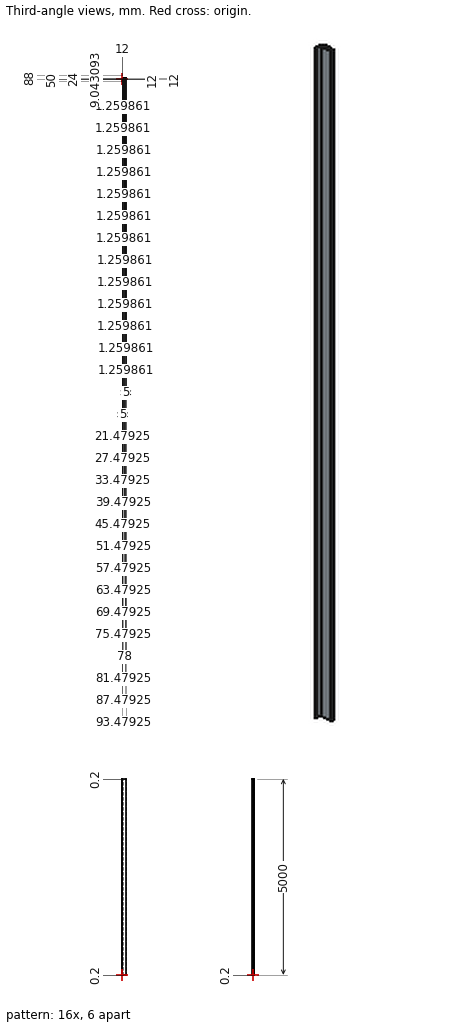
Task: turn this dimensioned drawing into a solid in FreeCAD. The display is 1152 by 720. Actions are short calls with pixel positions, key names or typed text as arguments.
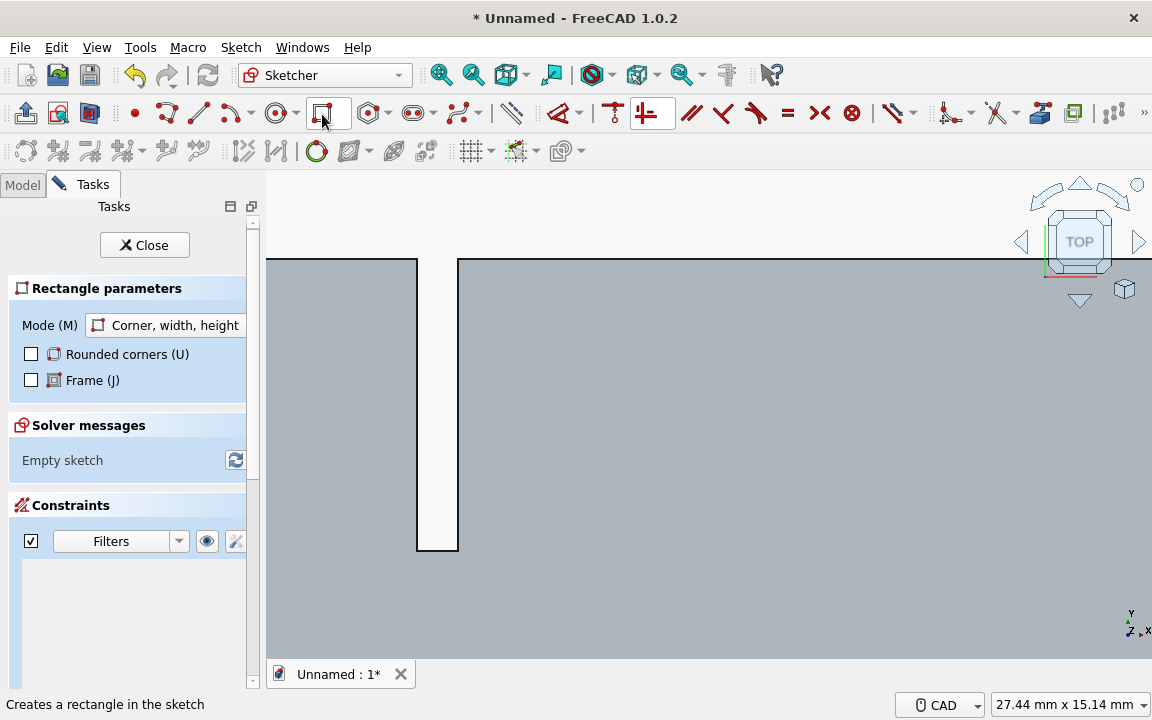
click(611, 259)
click(652, 551)
key(Escape)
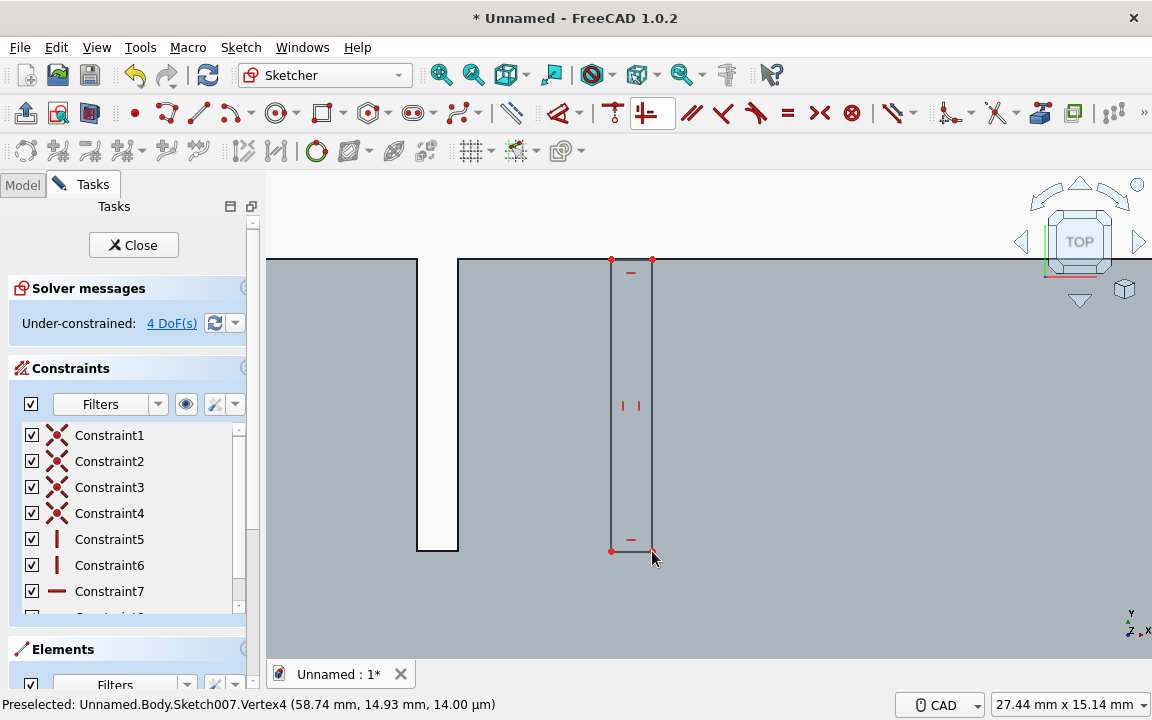
click(558, 114)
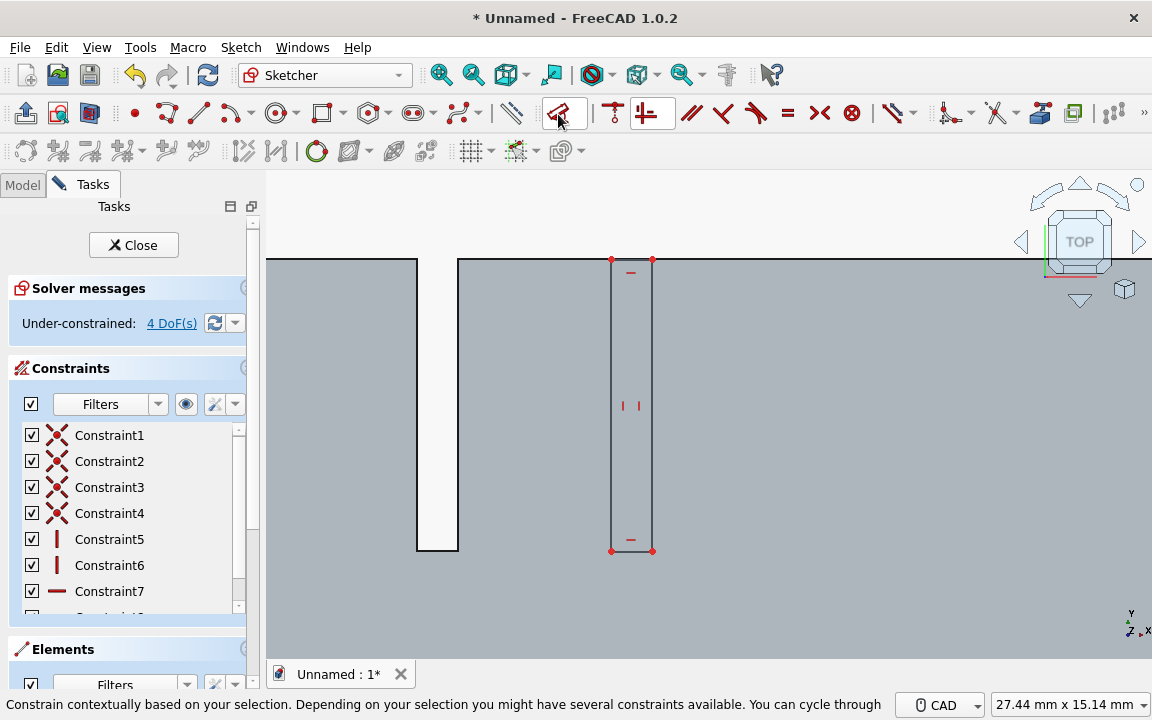
click(611, 260)
click(645, 575)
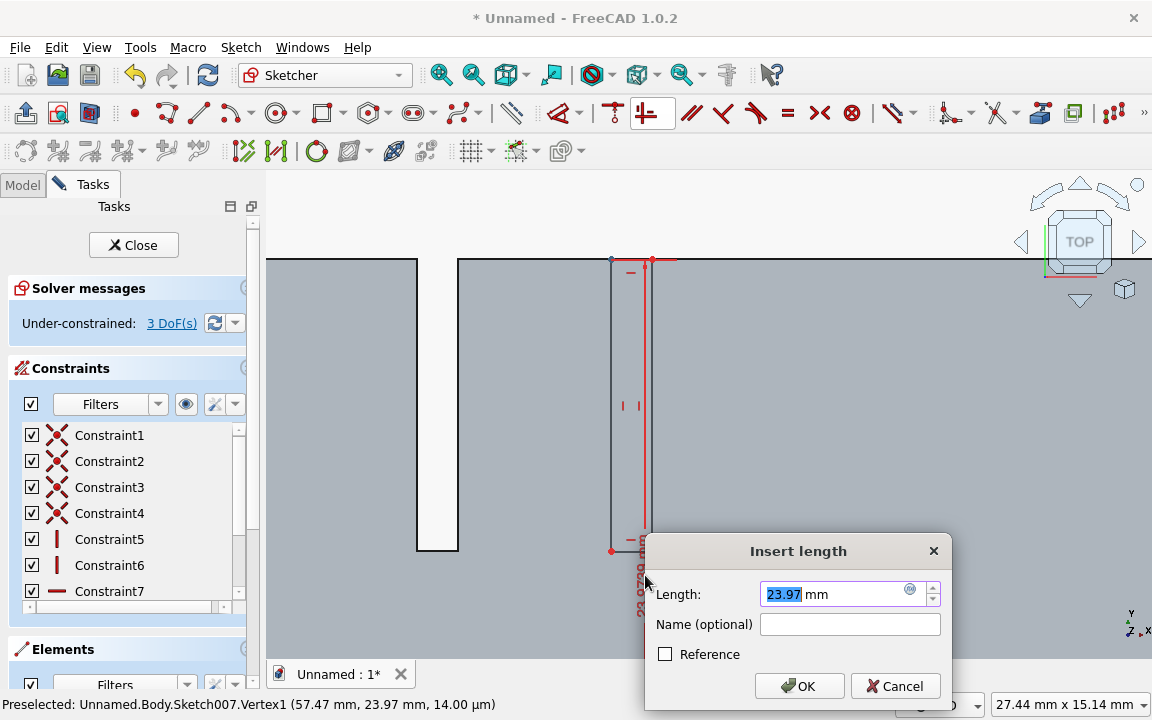
text(24)
key(Return)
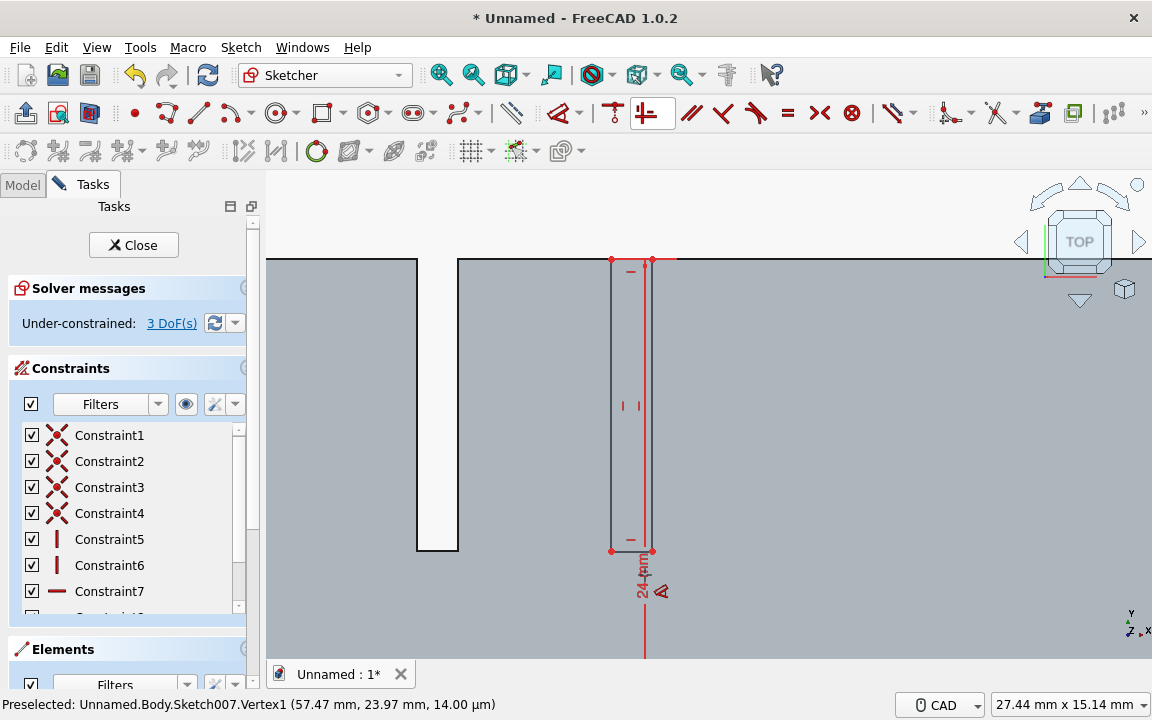
click(611, 347)
click(577, 406)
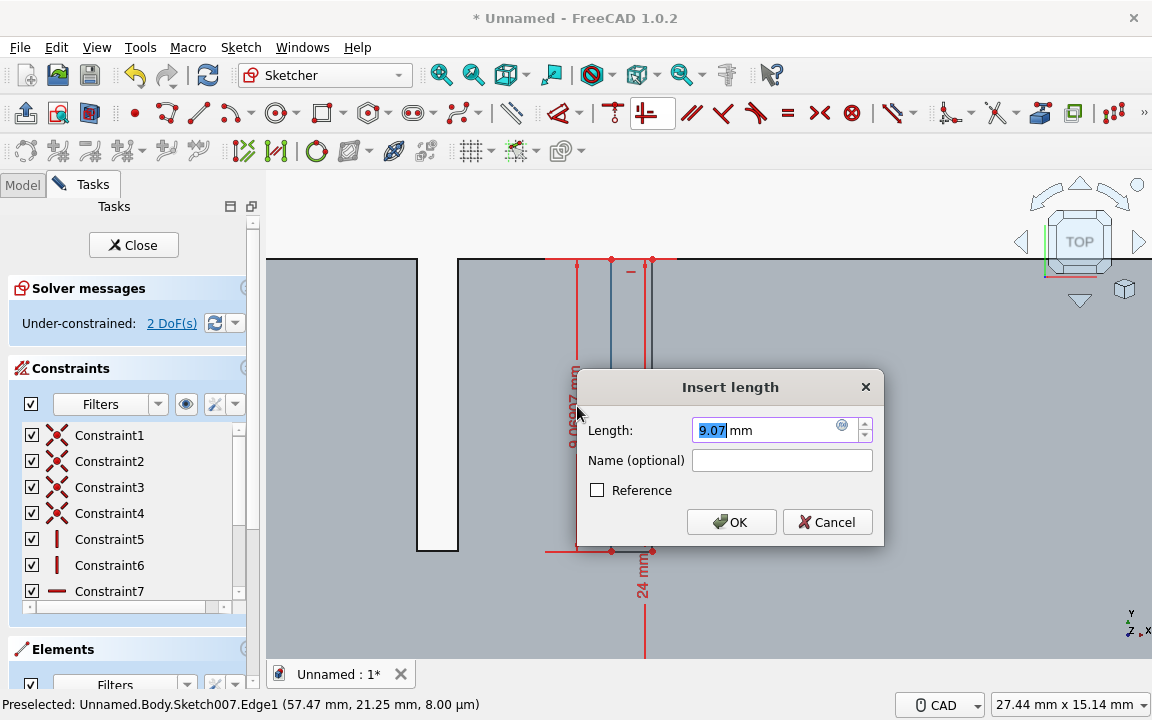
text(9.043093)
key(Return)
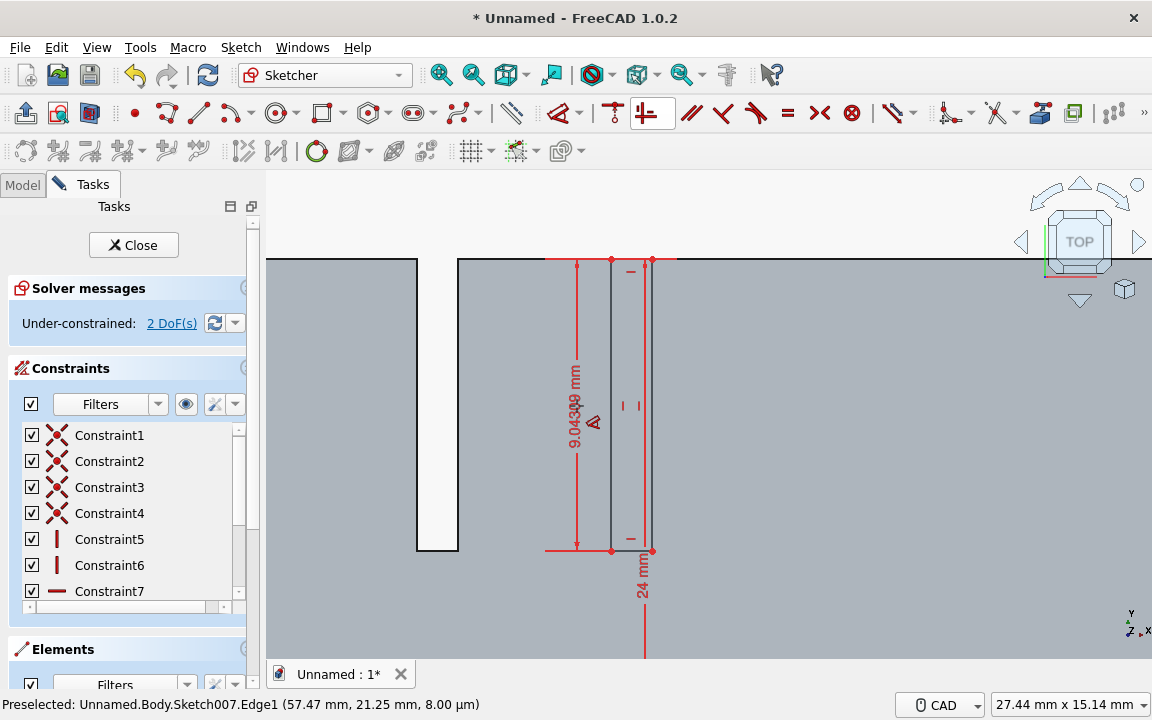
click(623, 551)
click(631, 517)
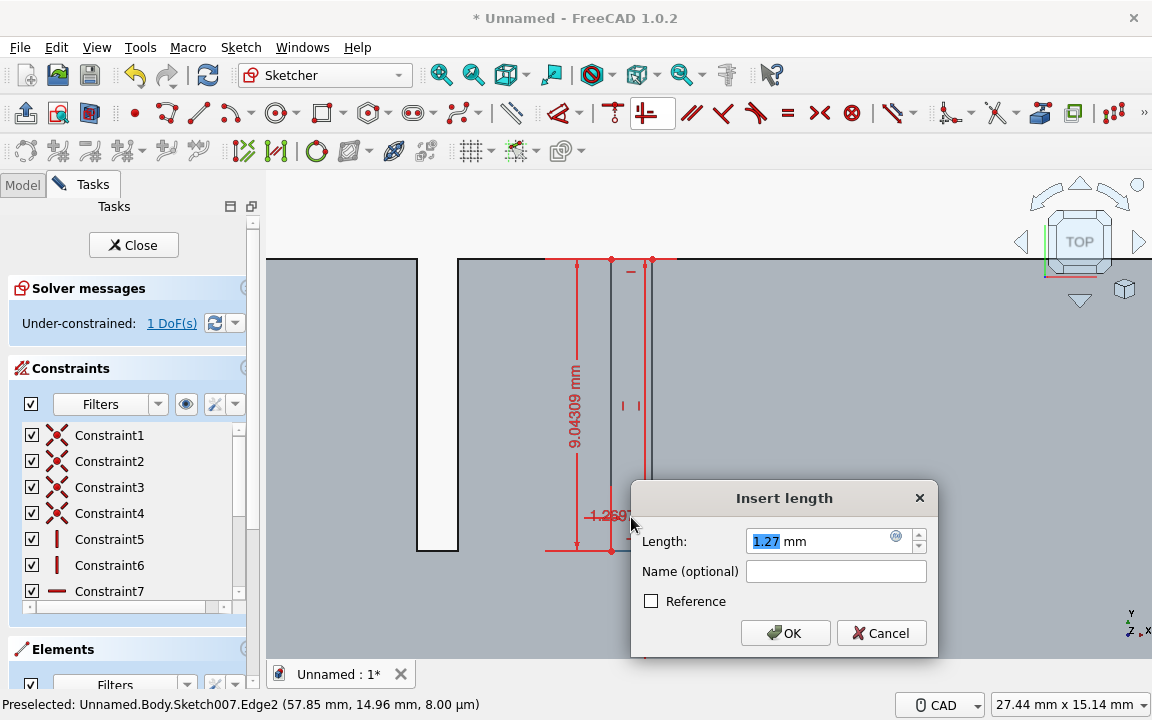
text(1.259861)
key(Return)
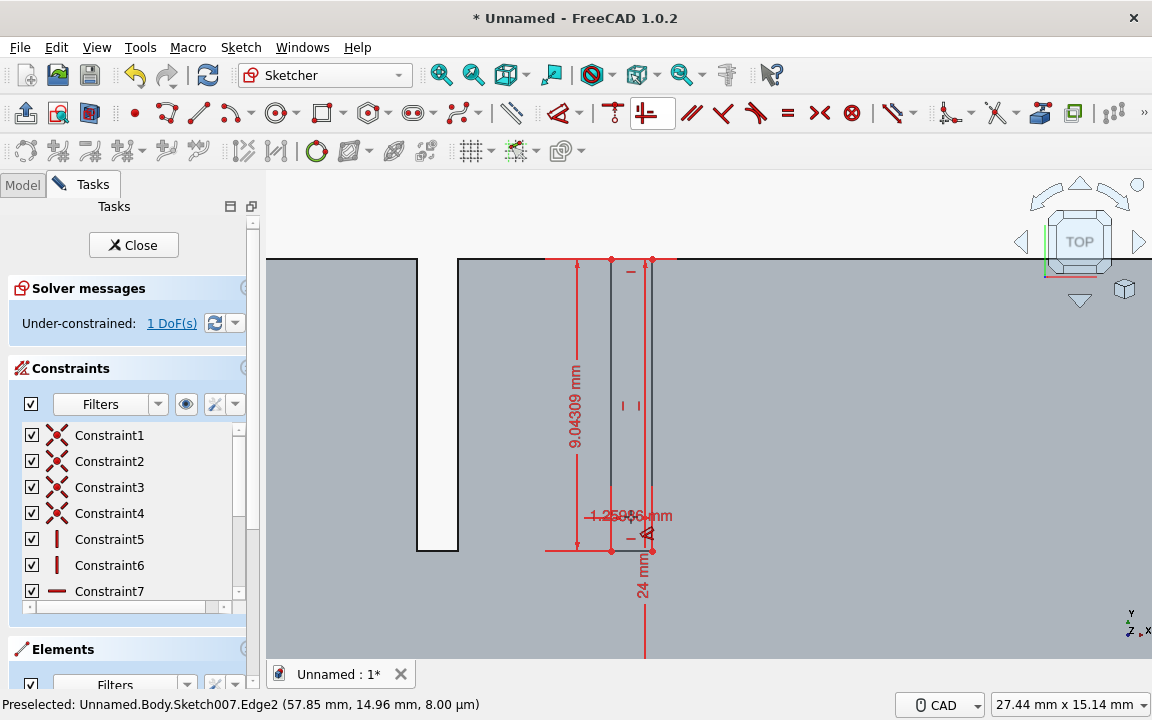
click(611, 259)
click(453, 225)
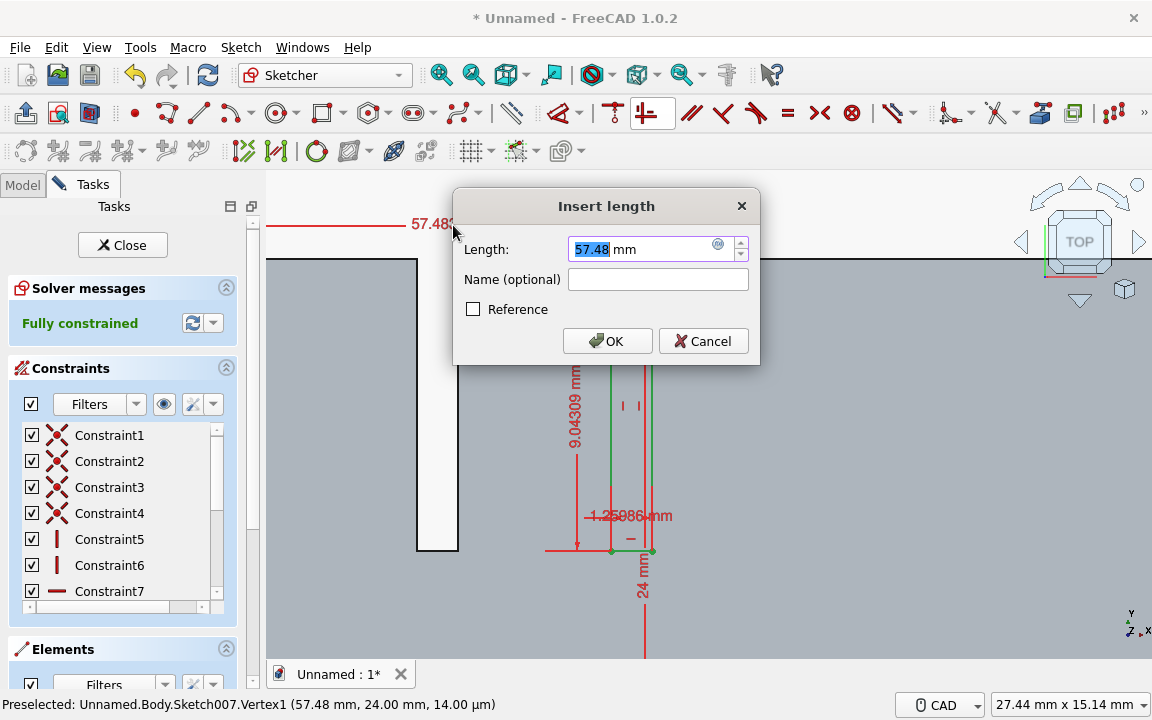
text(57.47925)
key(Return)
key(Escape)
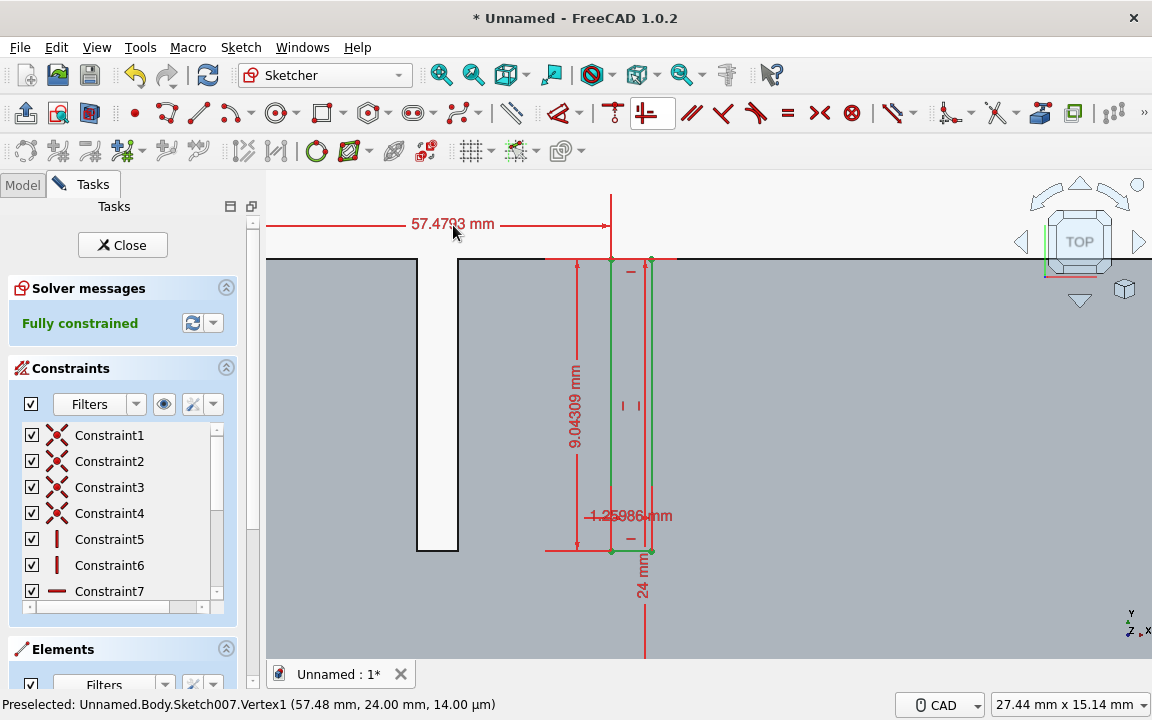
click(123, 245)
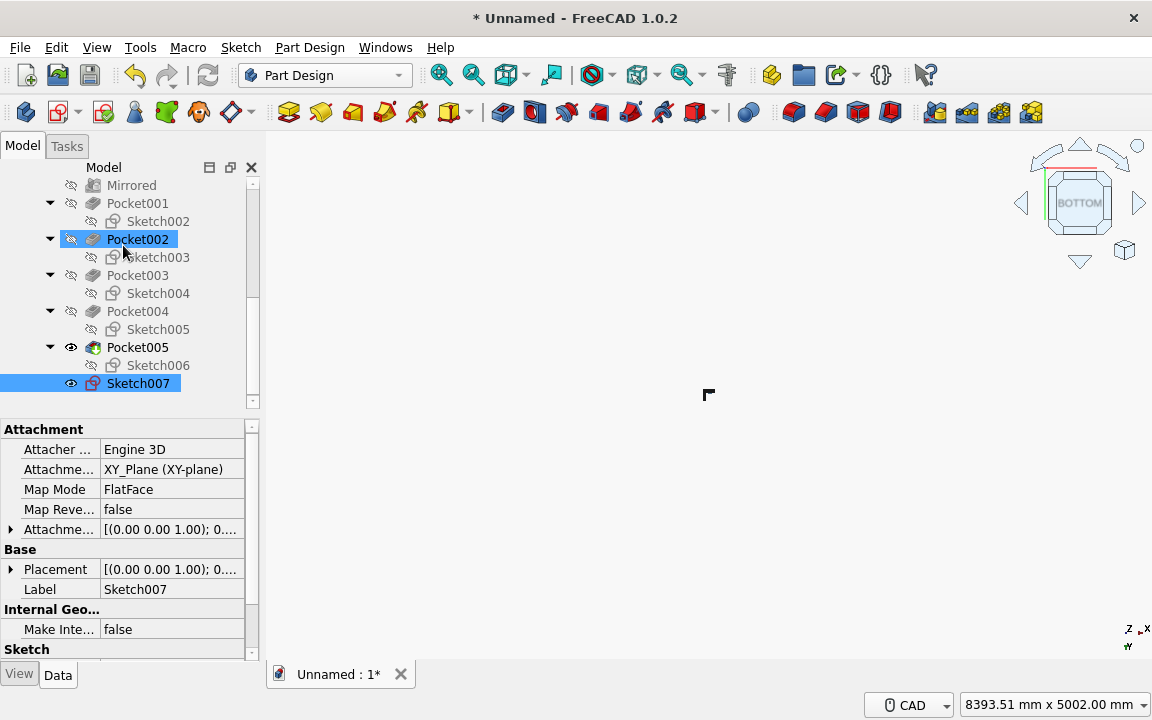
click(504, 112)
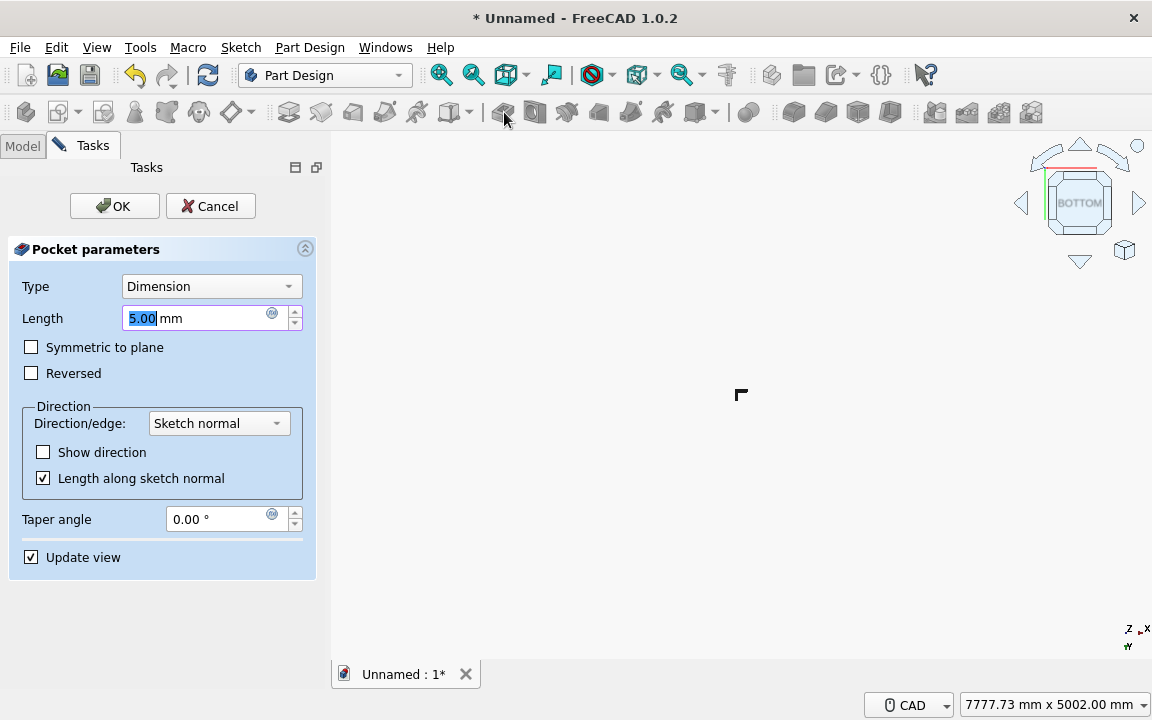
text(0.2)
key(Tab)